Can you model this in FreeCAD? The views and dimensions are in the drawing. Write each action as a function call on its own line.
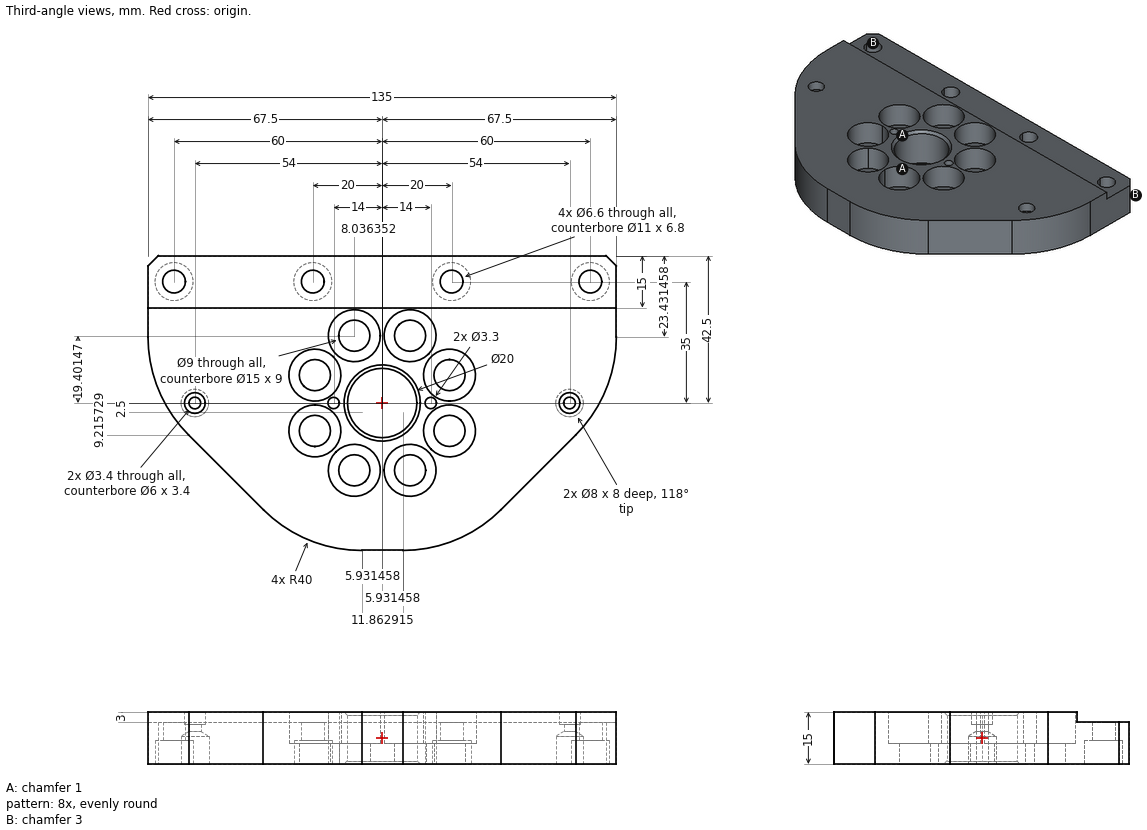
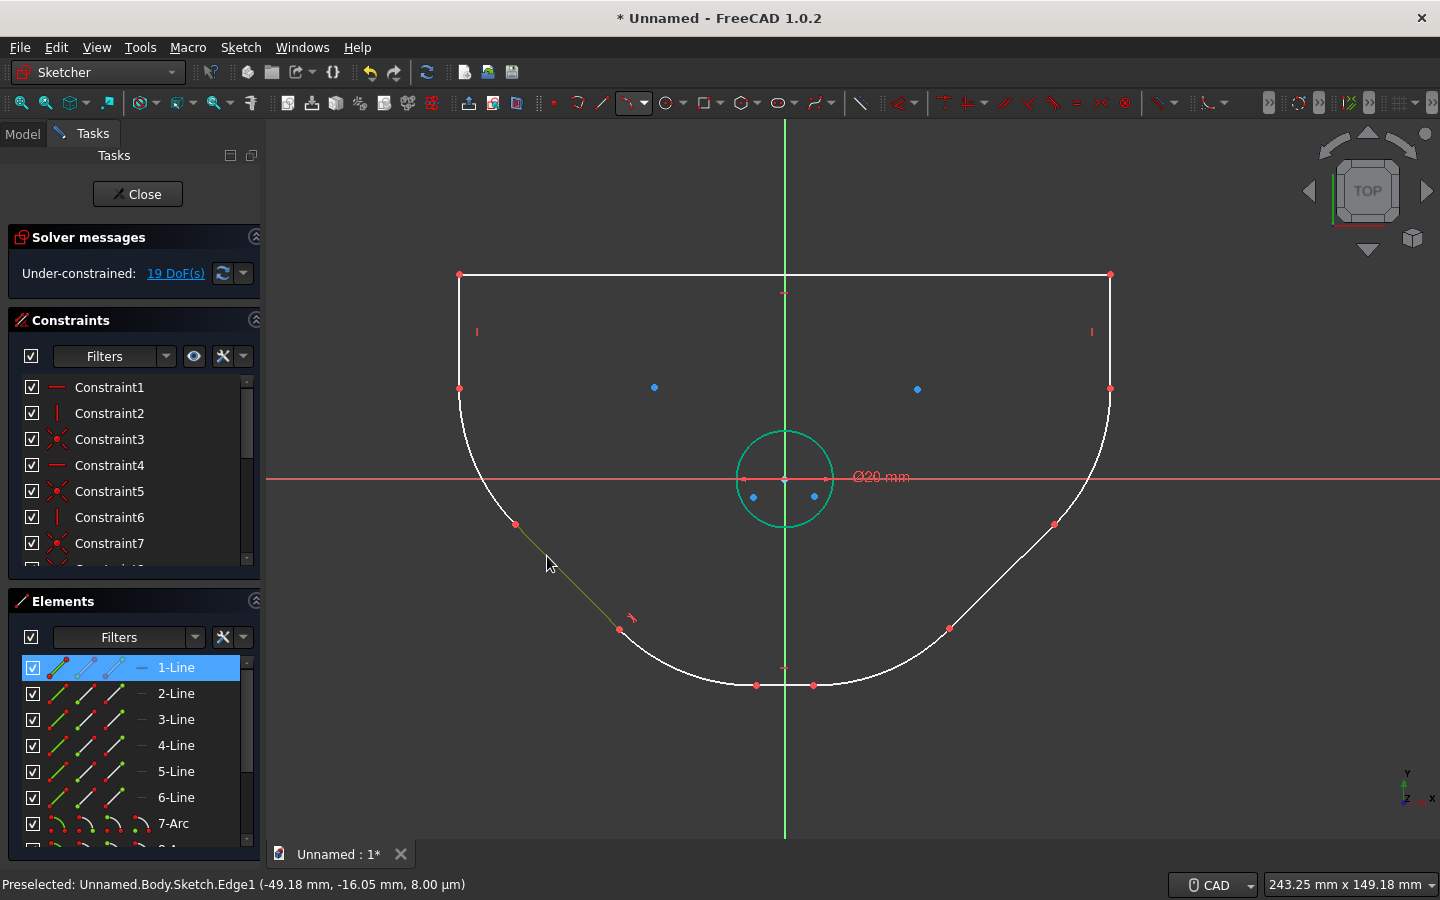
click(465, 433)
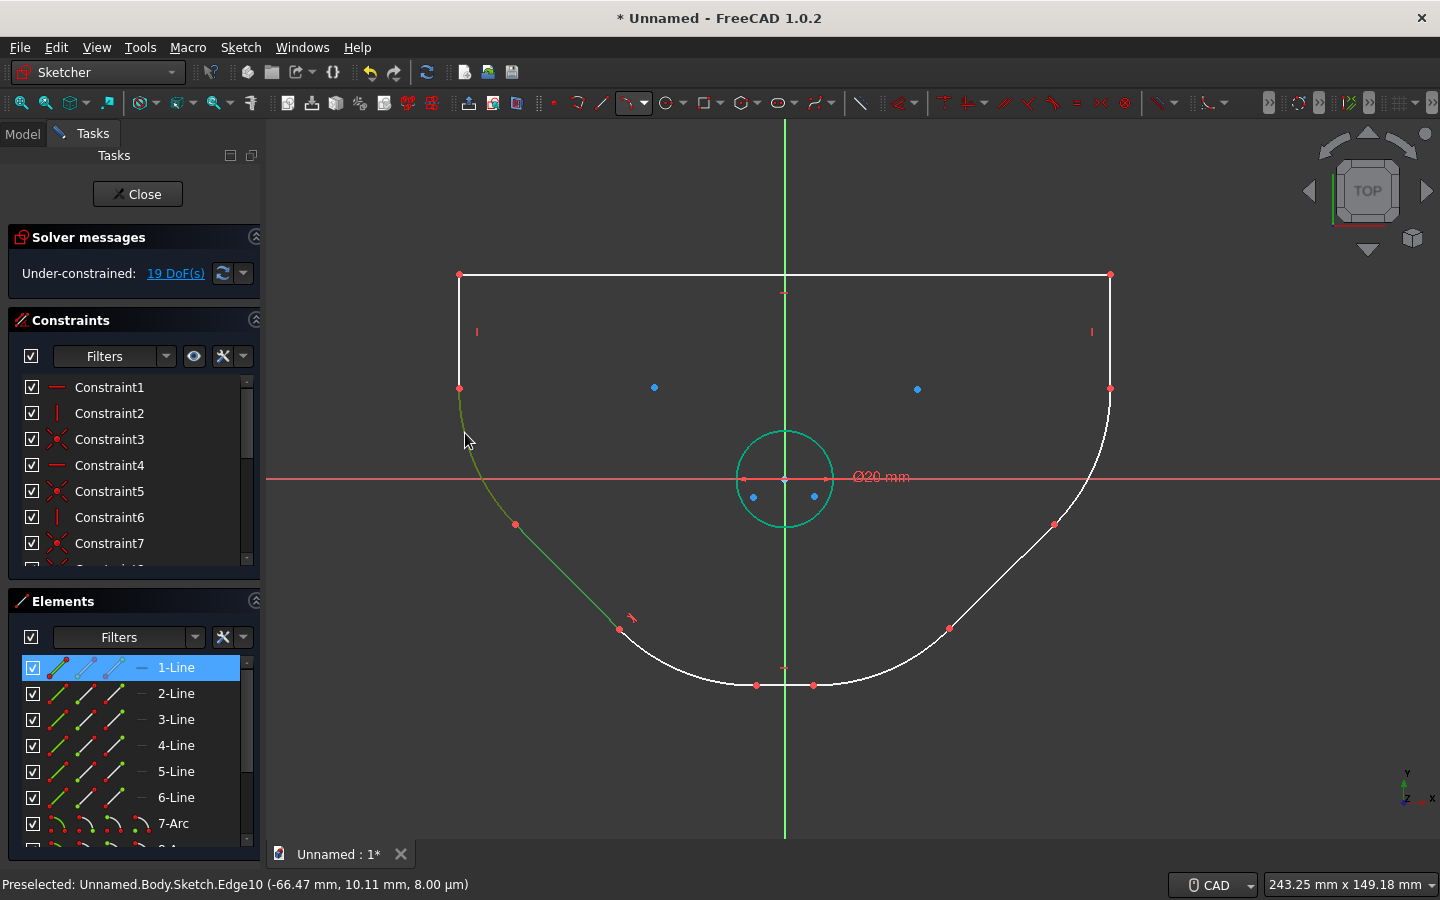
click(1054, 104)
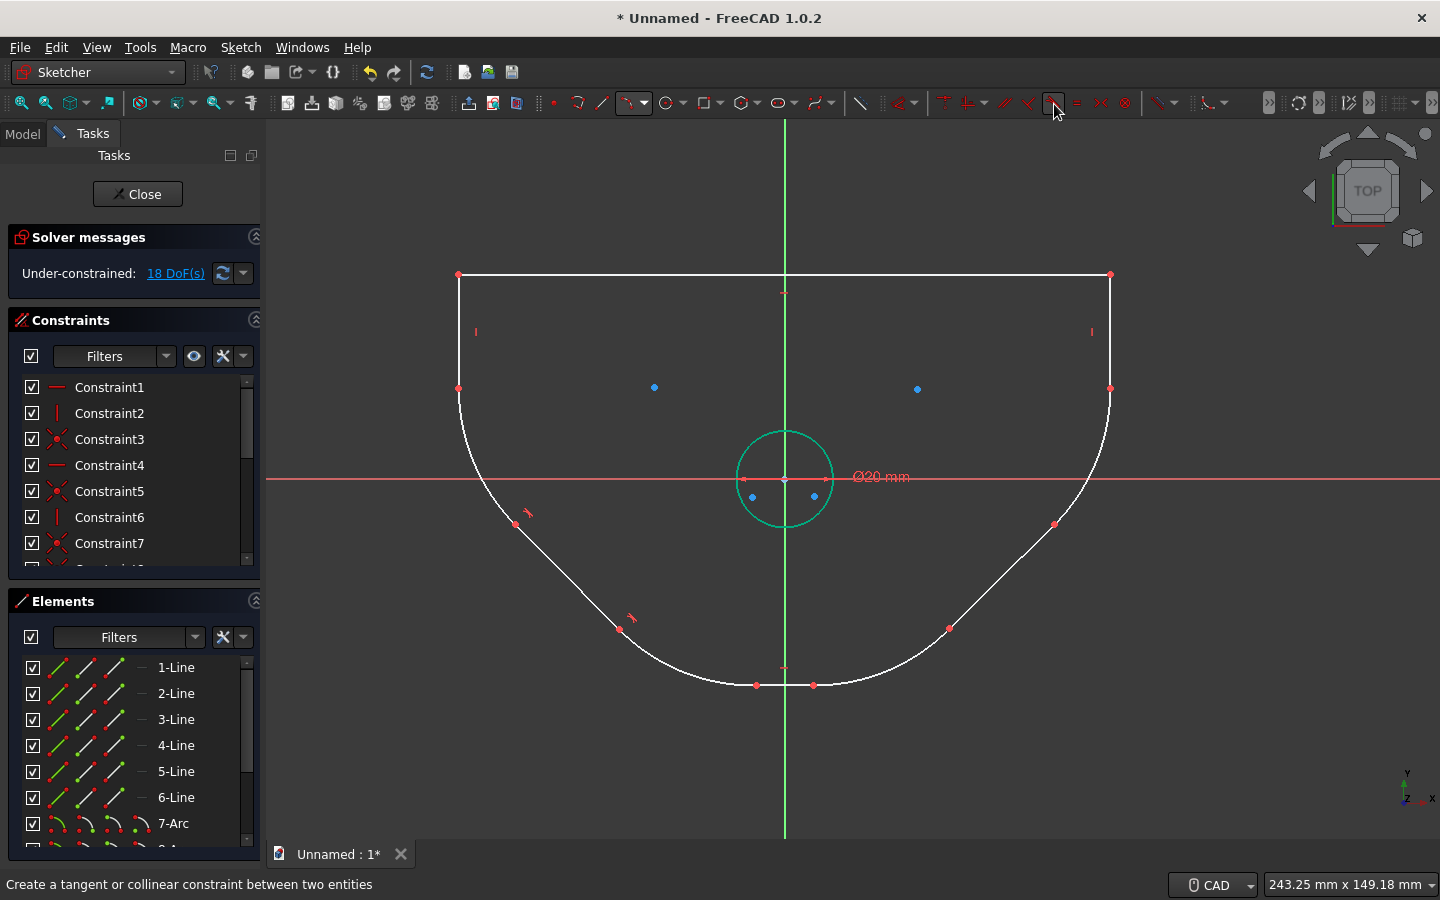
click(981, 597)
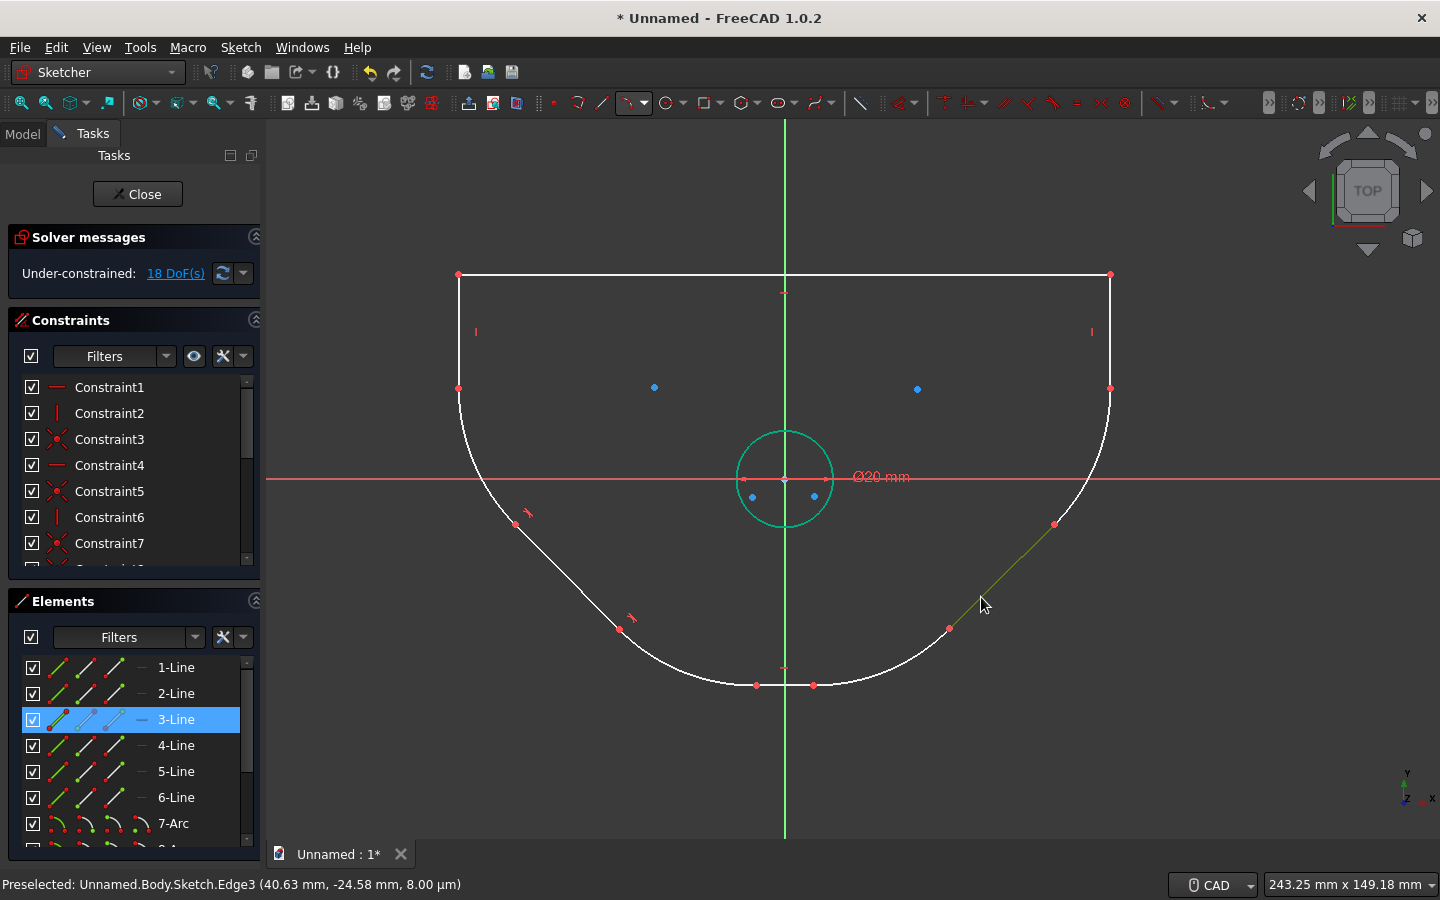
click(858, 680)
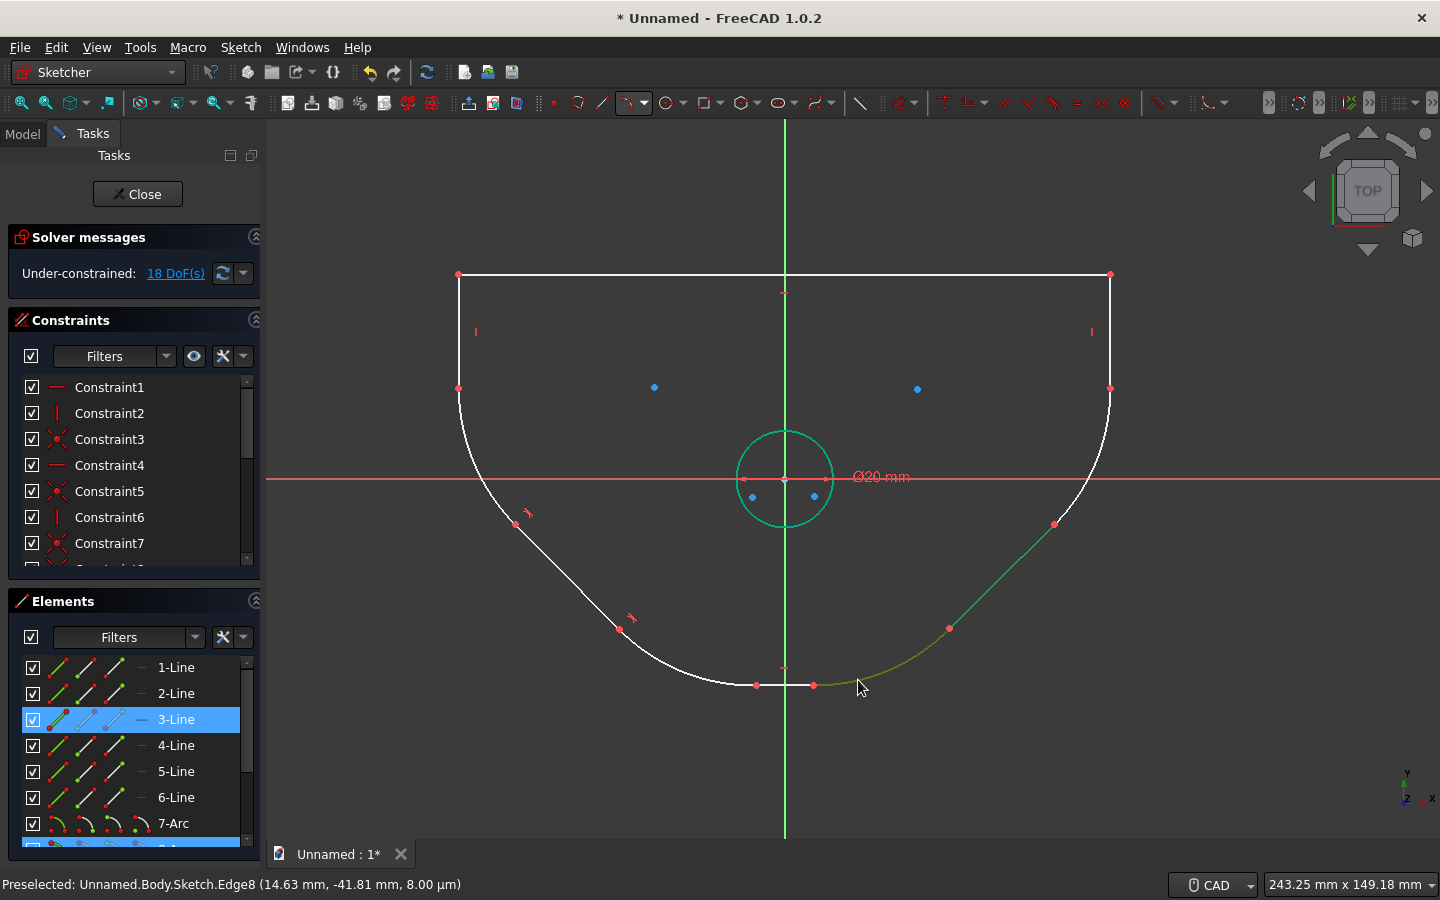
click(1054, 104)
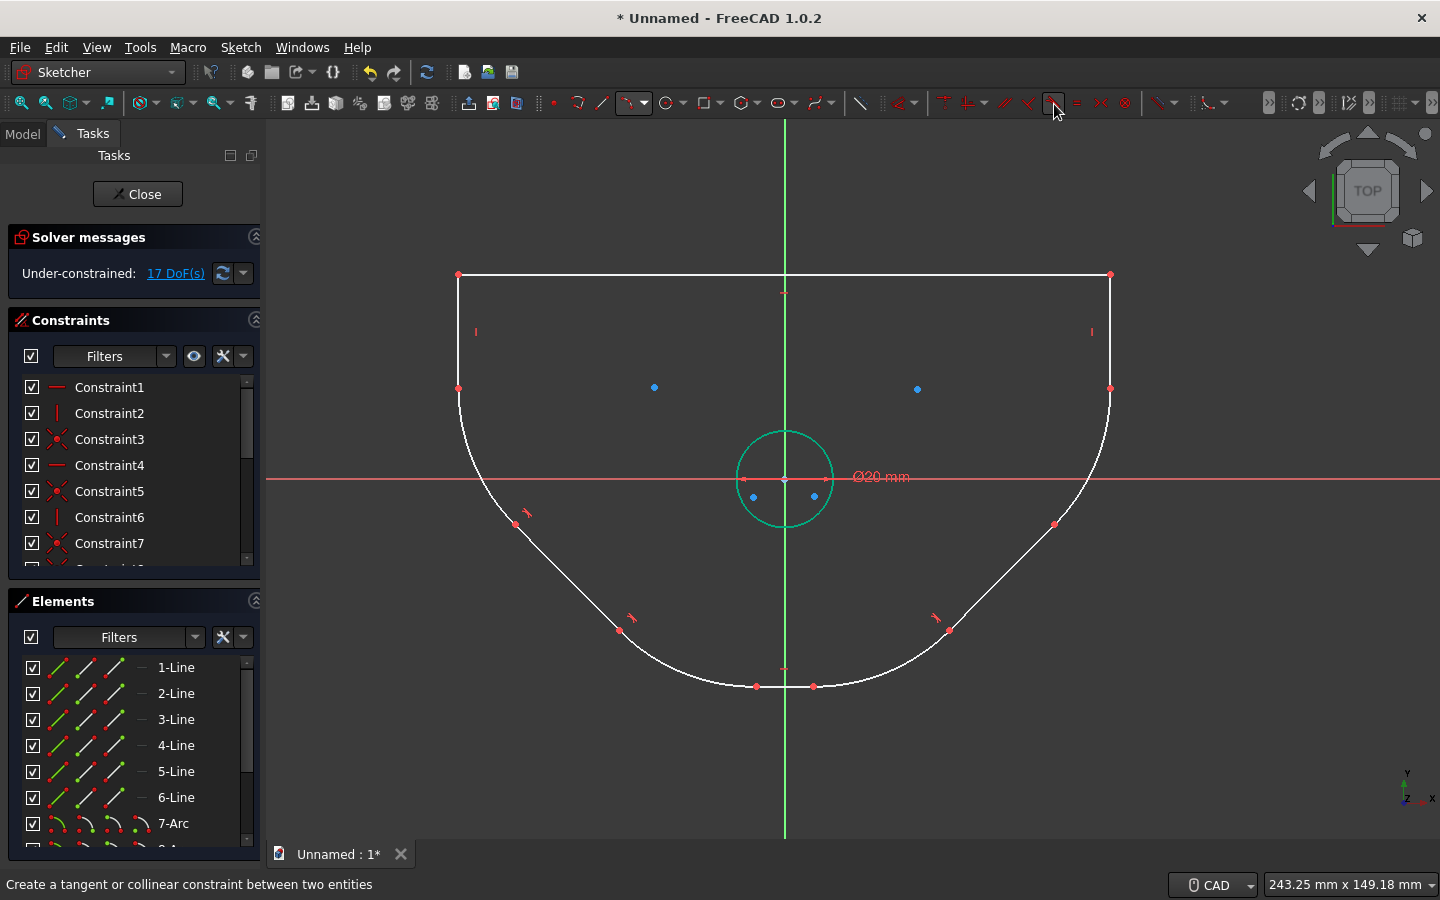
click(981, 599)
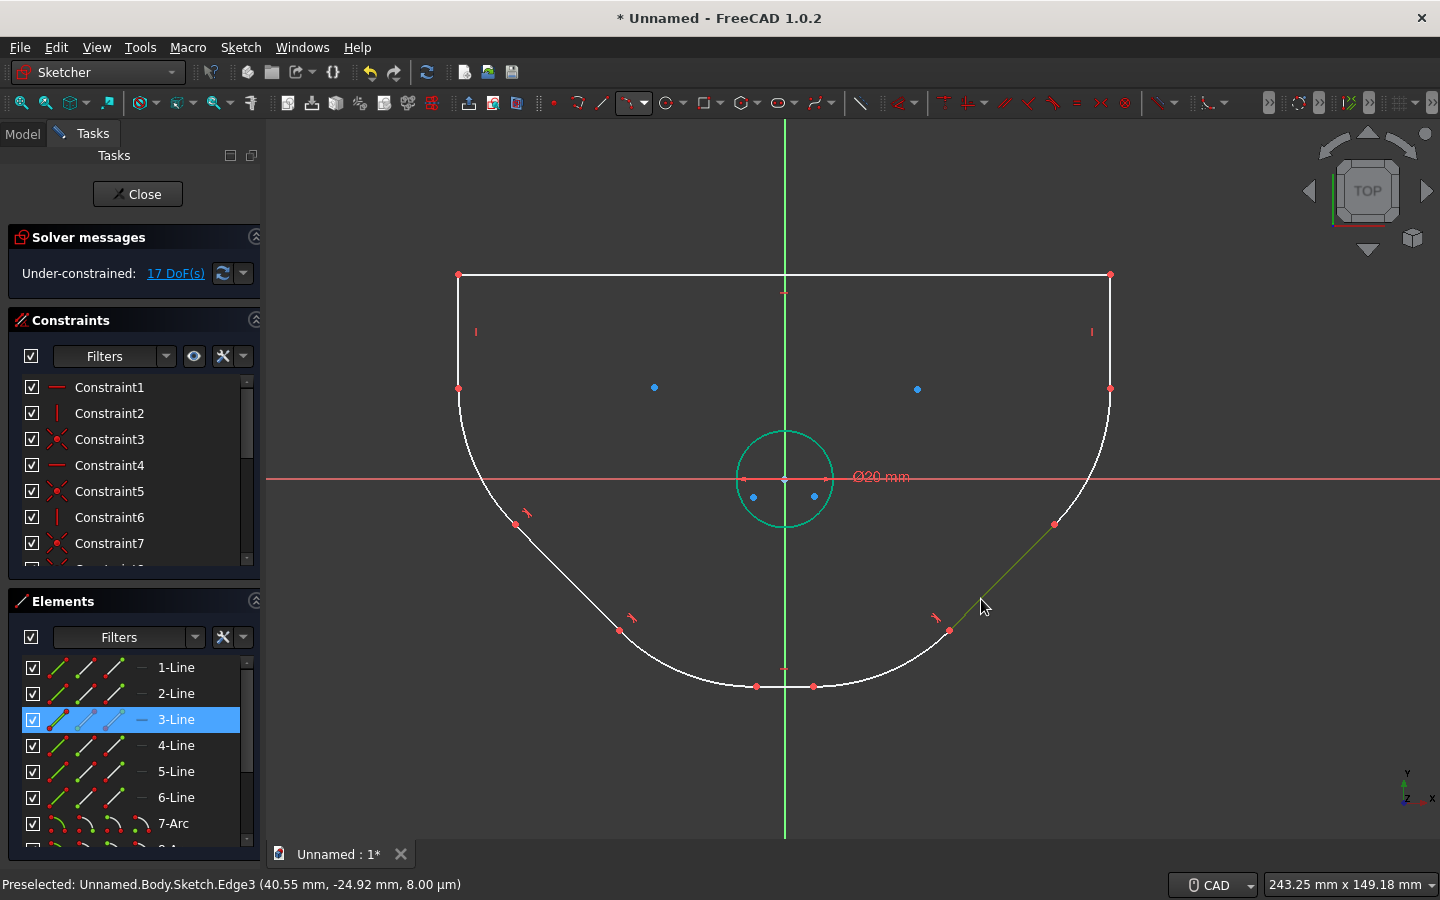
scroll(1082, 489, up, 2)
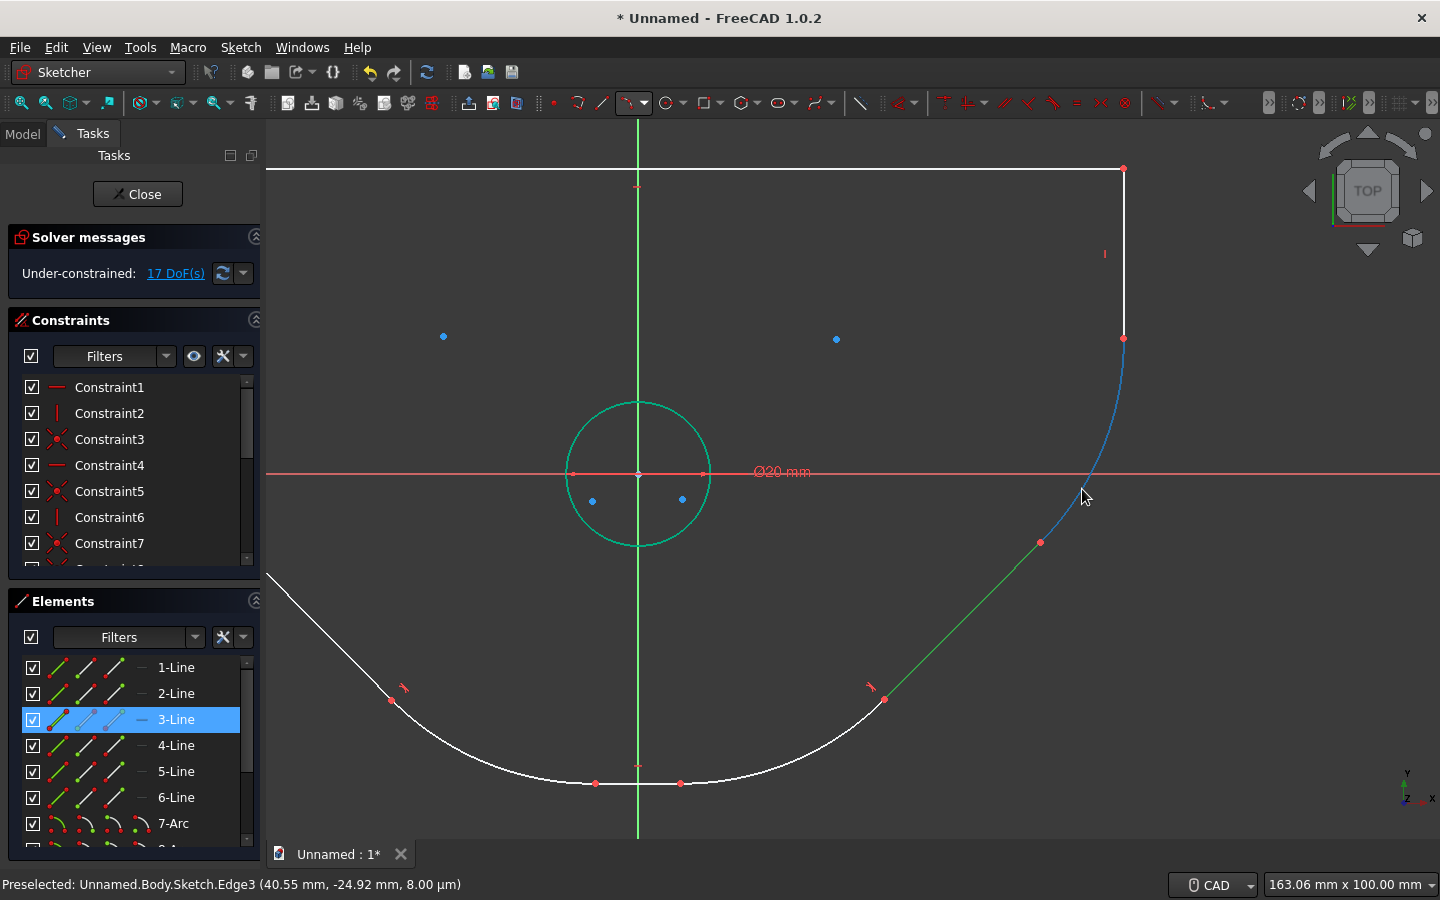
click(1082, 489)